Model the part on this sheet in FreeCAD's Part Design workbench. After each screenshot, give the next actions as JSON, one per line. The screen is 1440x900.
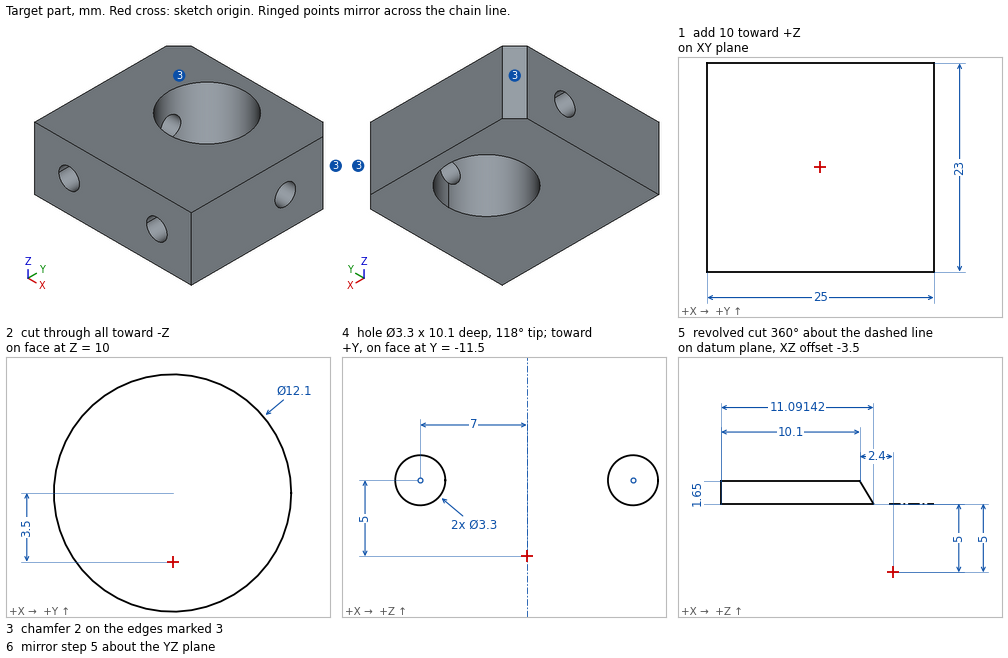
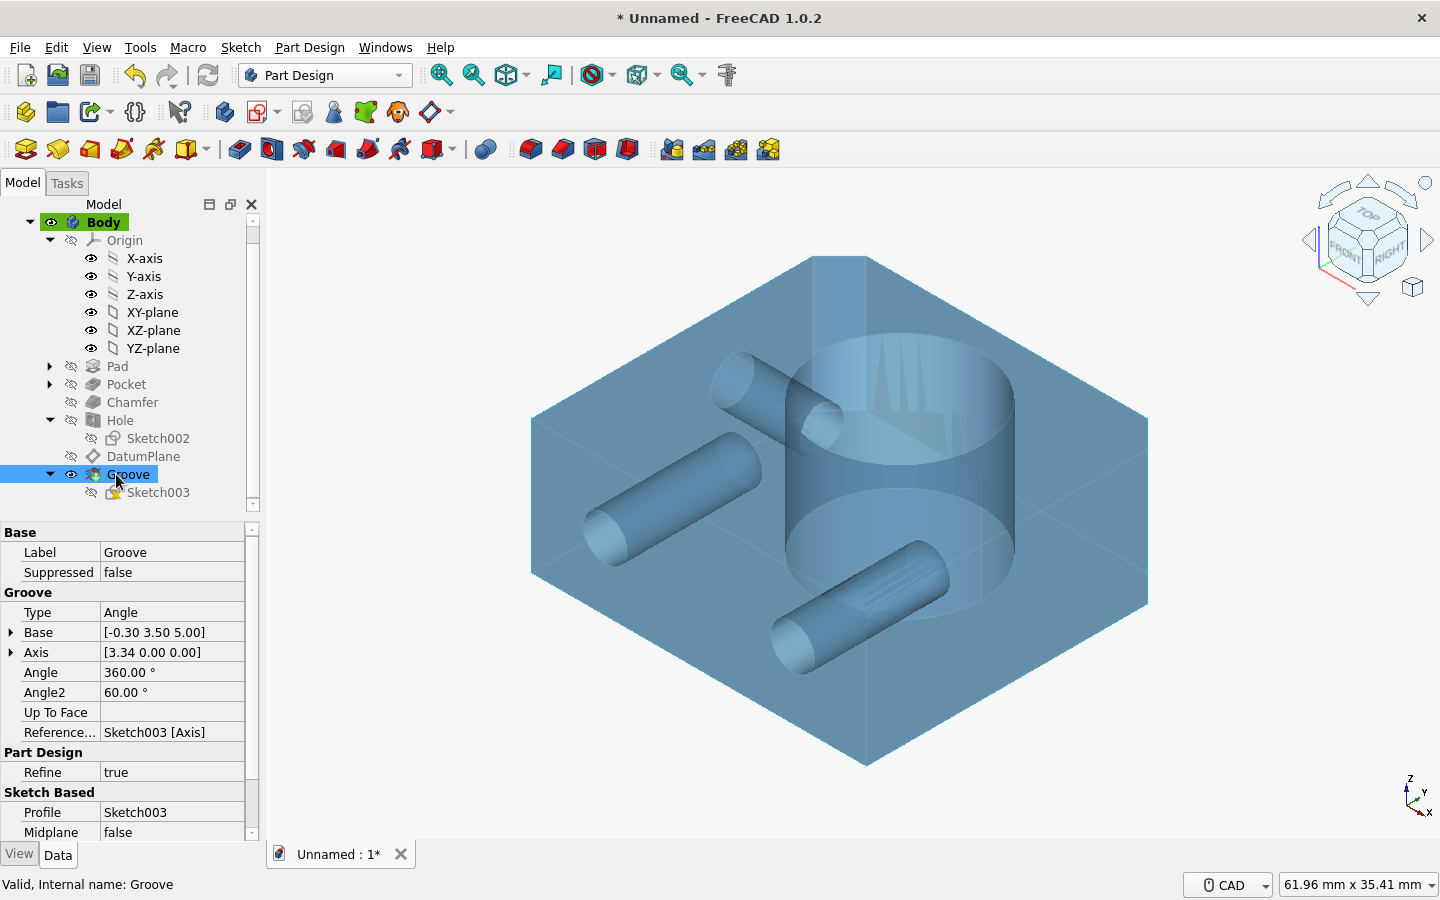
{"action": "left_click", "coordinate": [672, 150]}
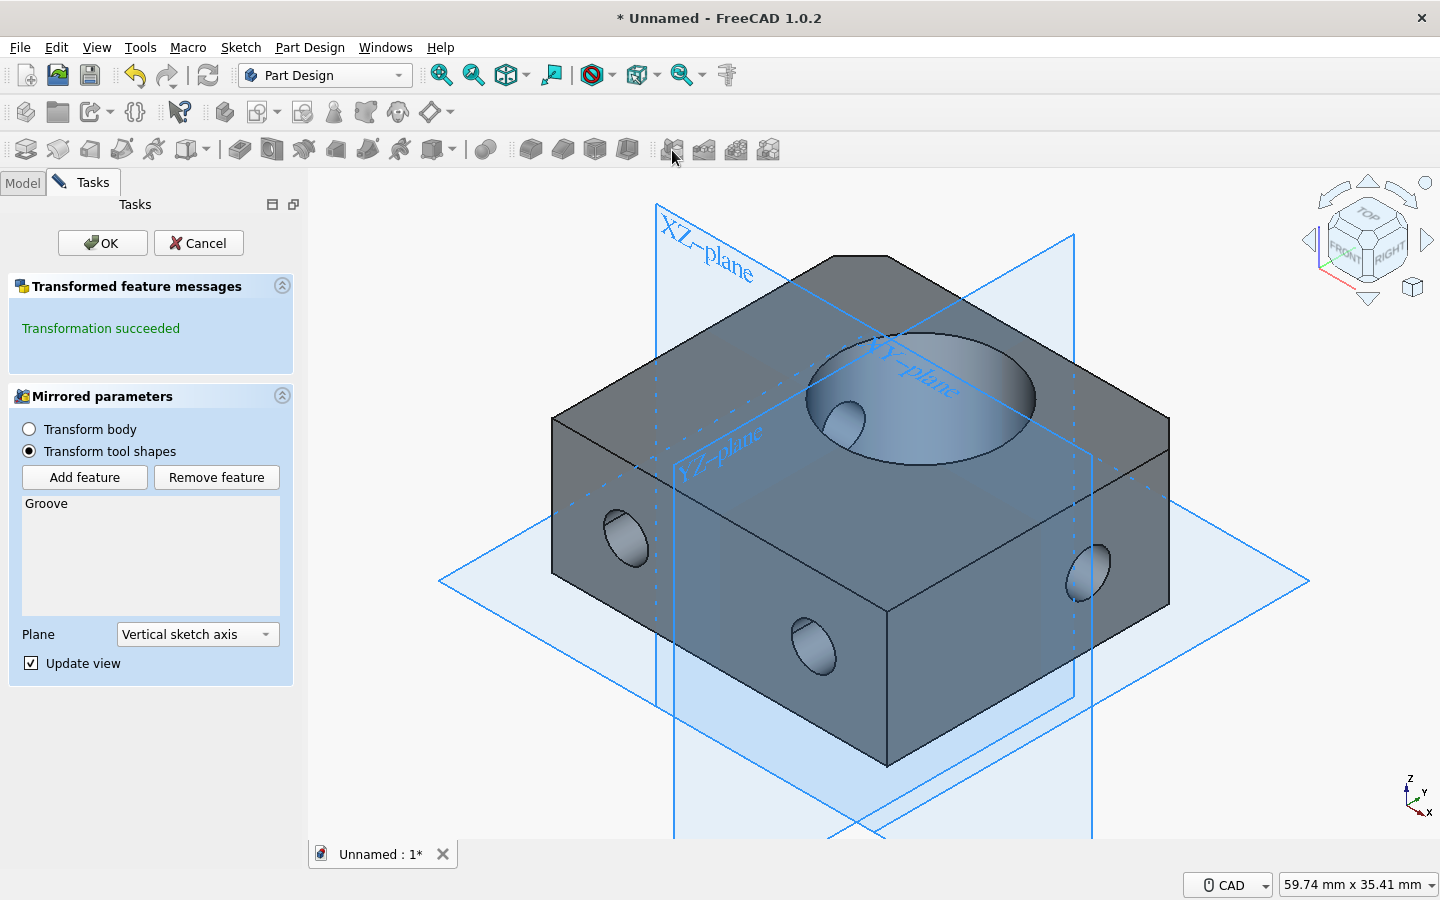
{"action": "left_click", "coordinate": [198, 634]}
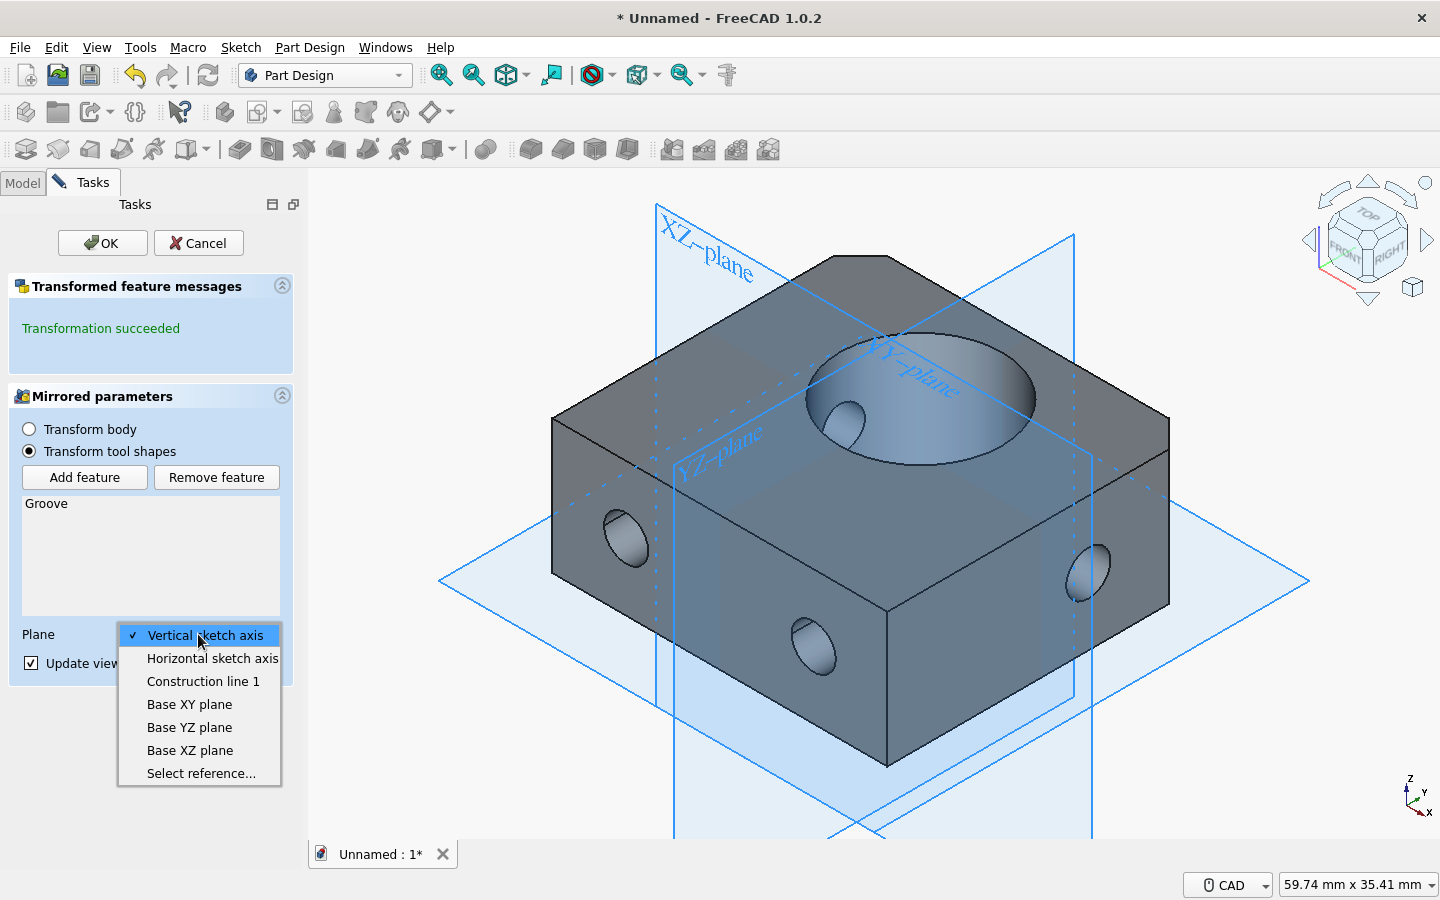
{"action": "left_click", "coordinate": [198, 728]}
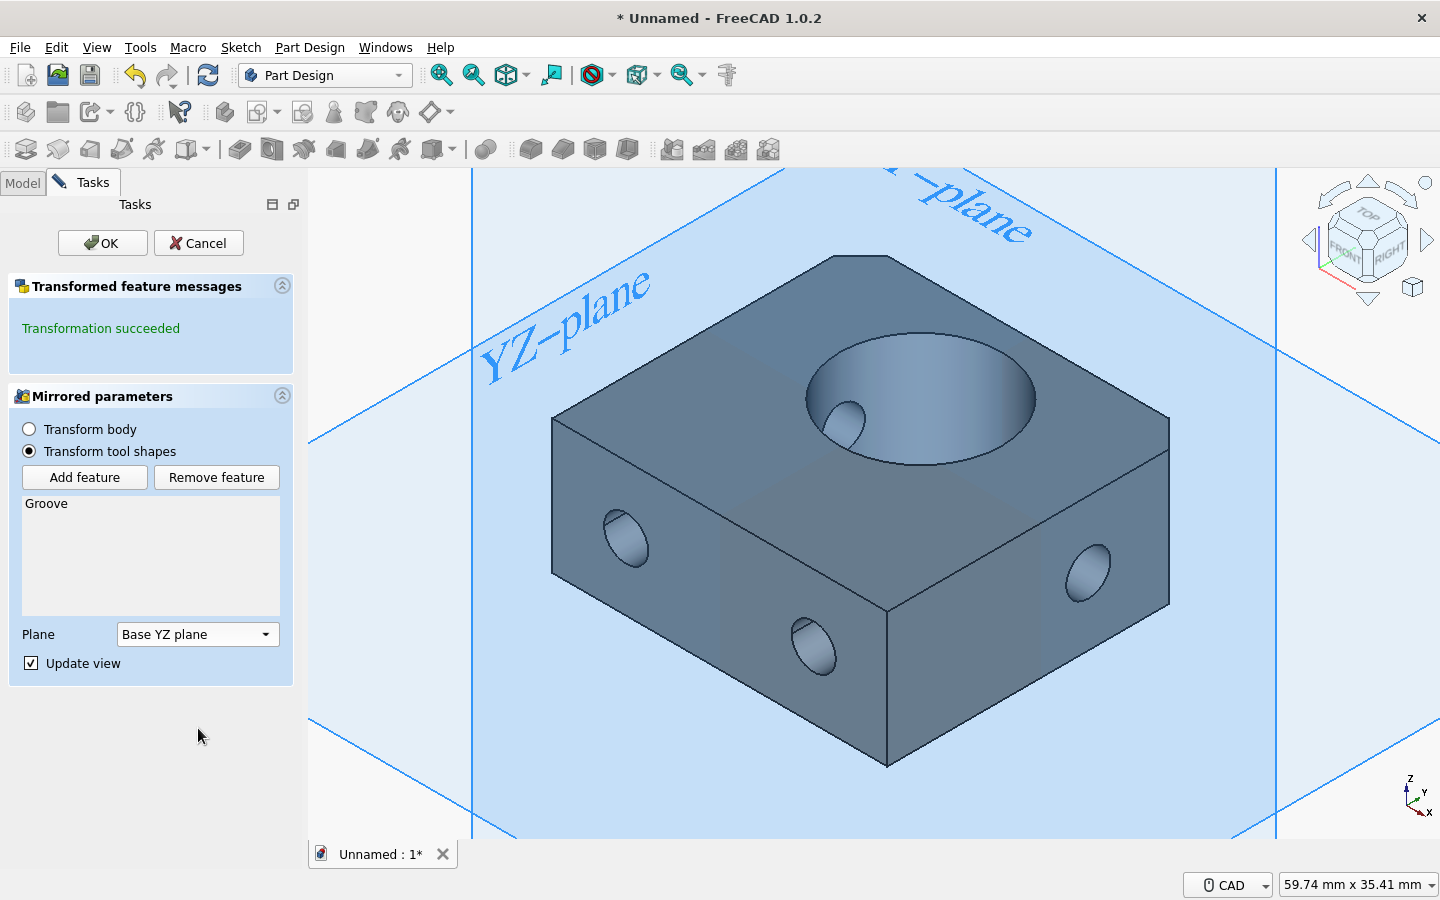
{"action": "left_click", "coordinate": [103, 243]}